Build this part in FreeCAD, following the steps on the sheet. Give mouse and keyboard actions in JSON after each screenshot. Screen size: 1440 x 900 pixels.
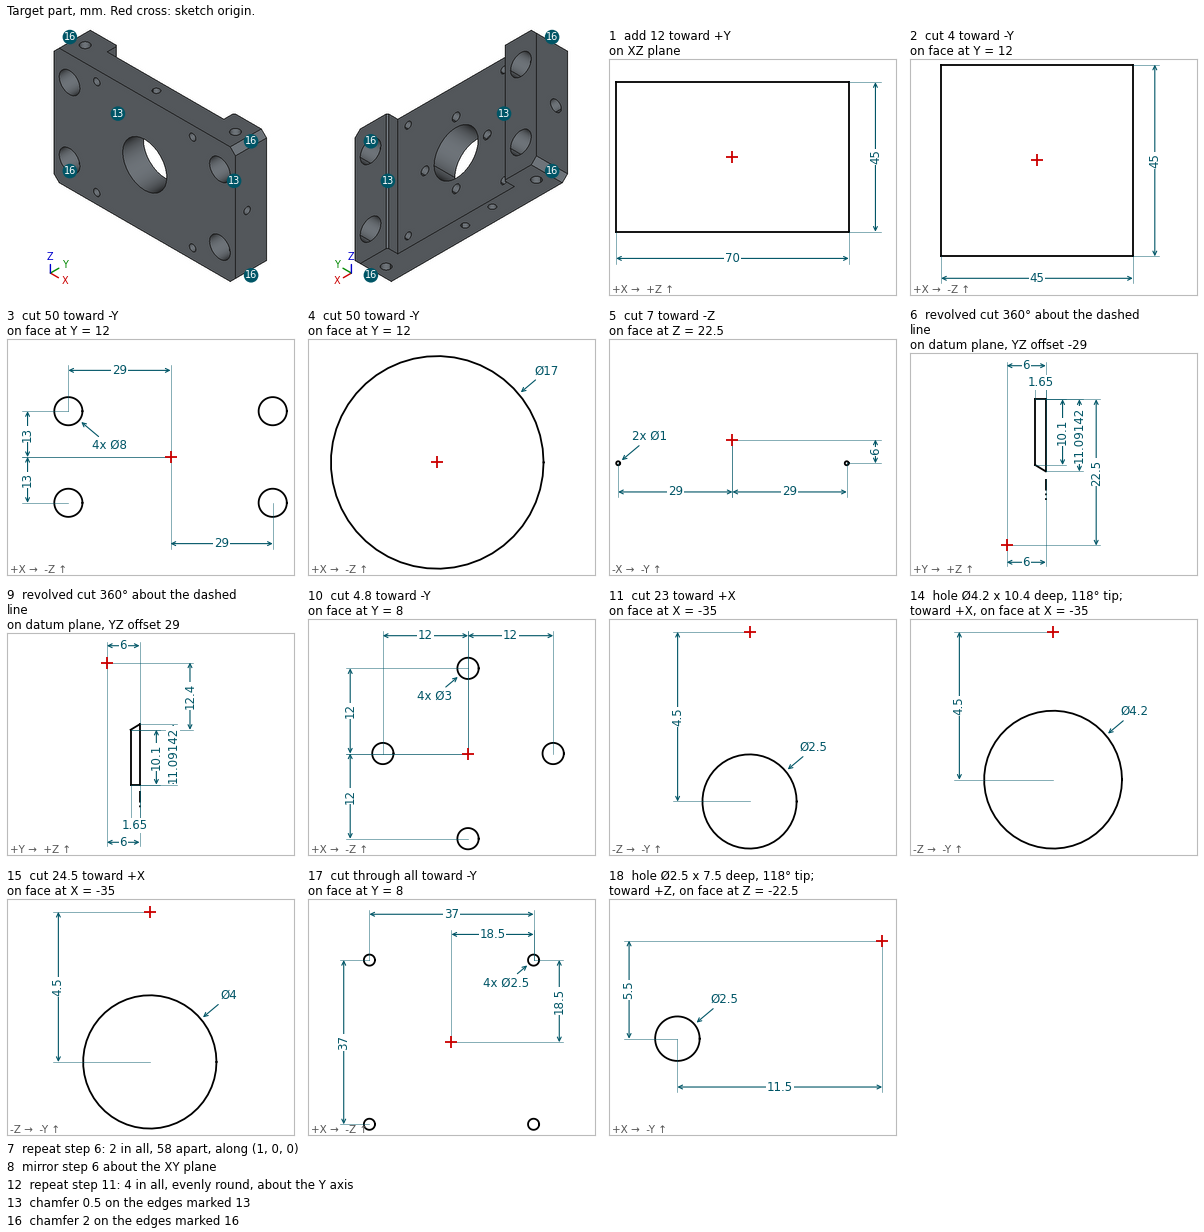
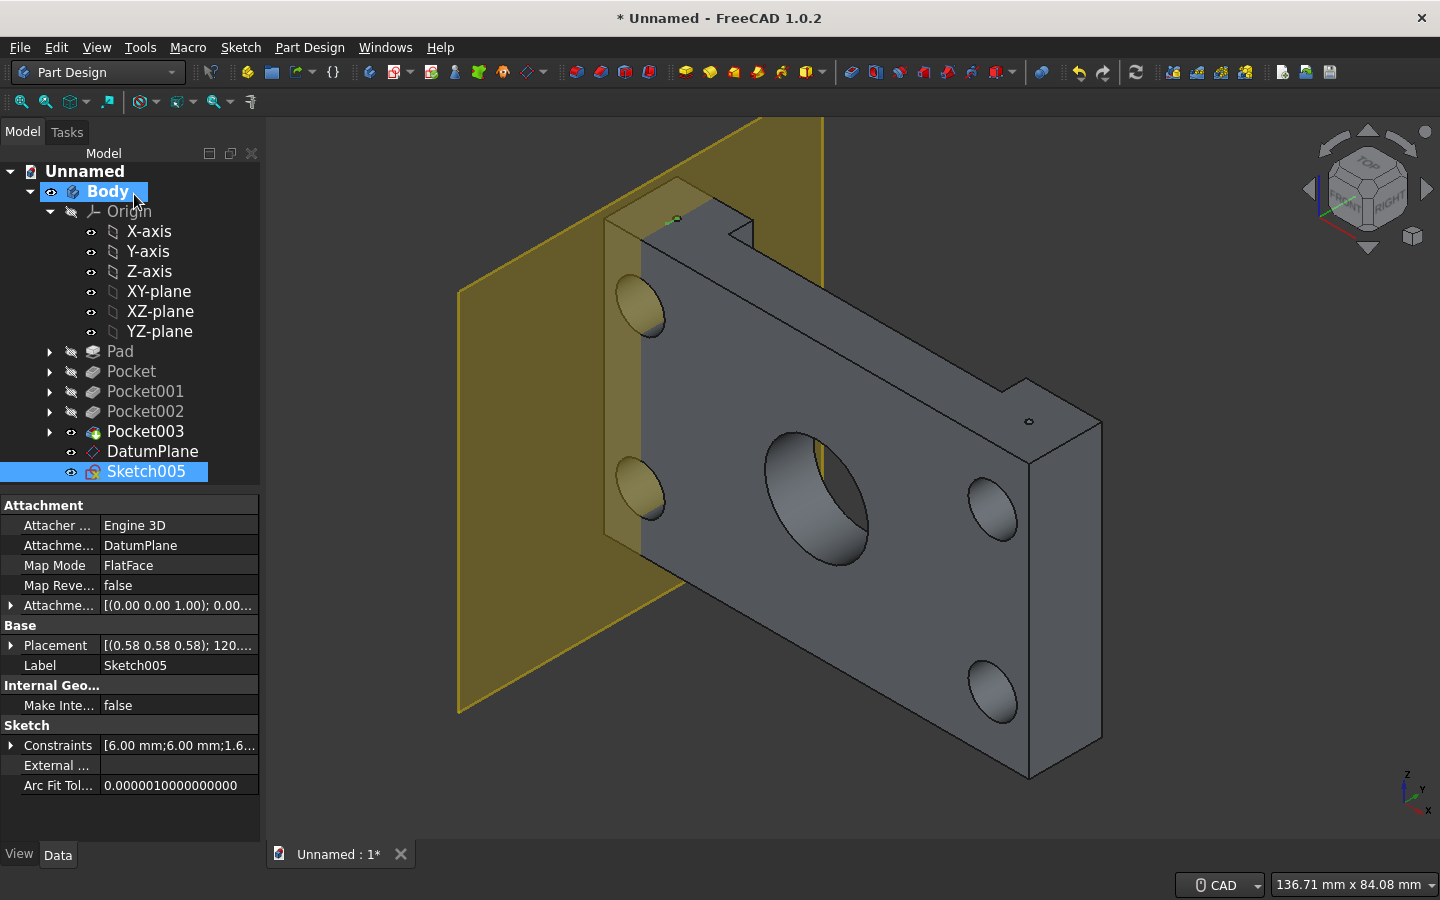
{"action": "left_click", "coordinate": [900, 72]}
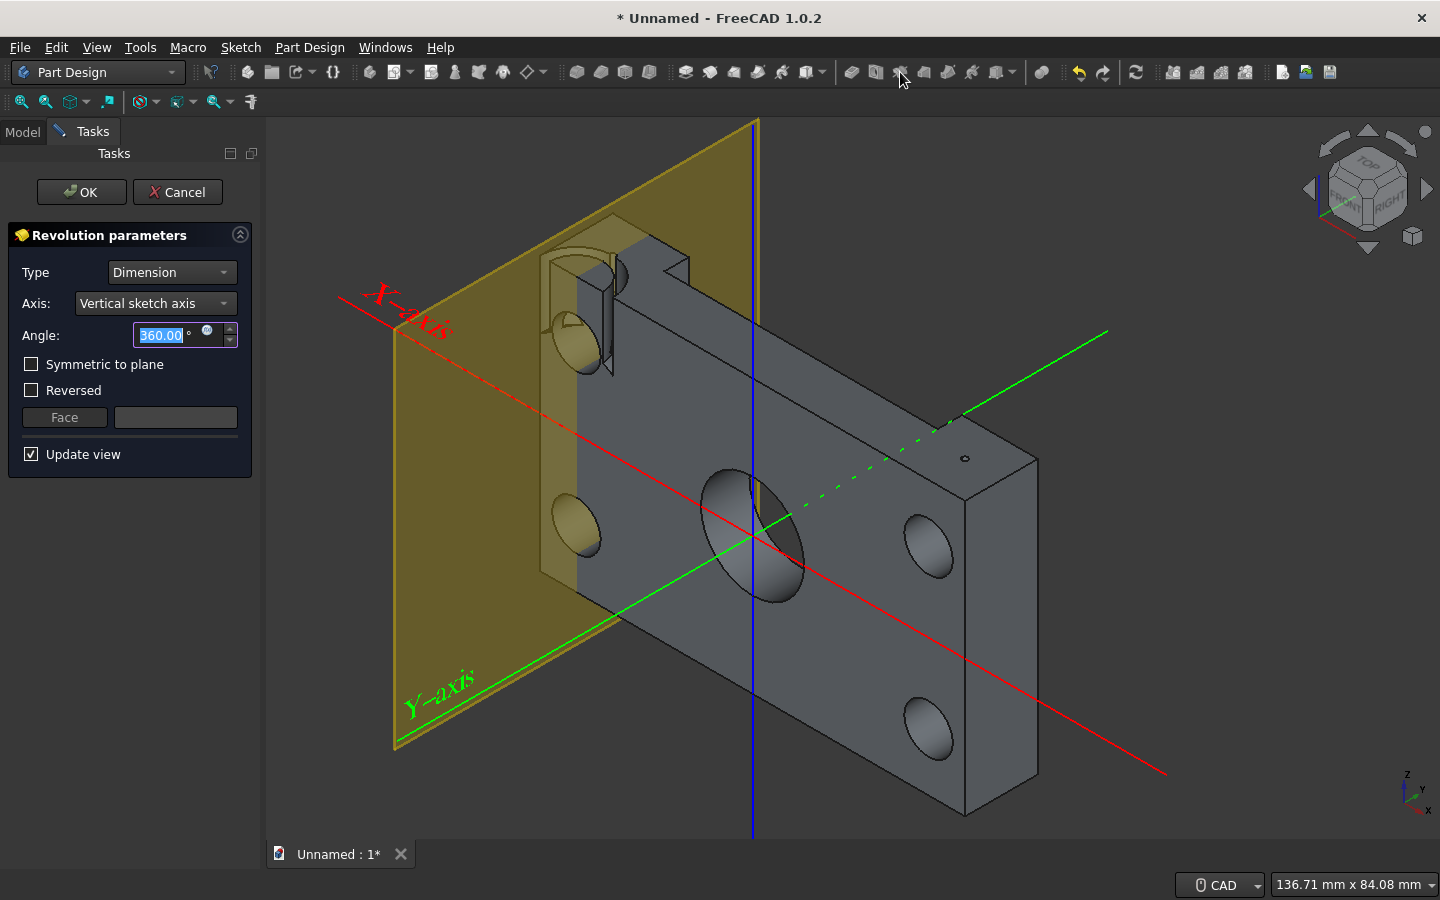
{"action": "left_click", "coordinate": [156, 304]}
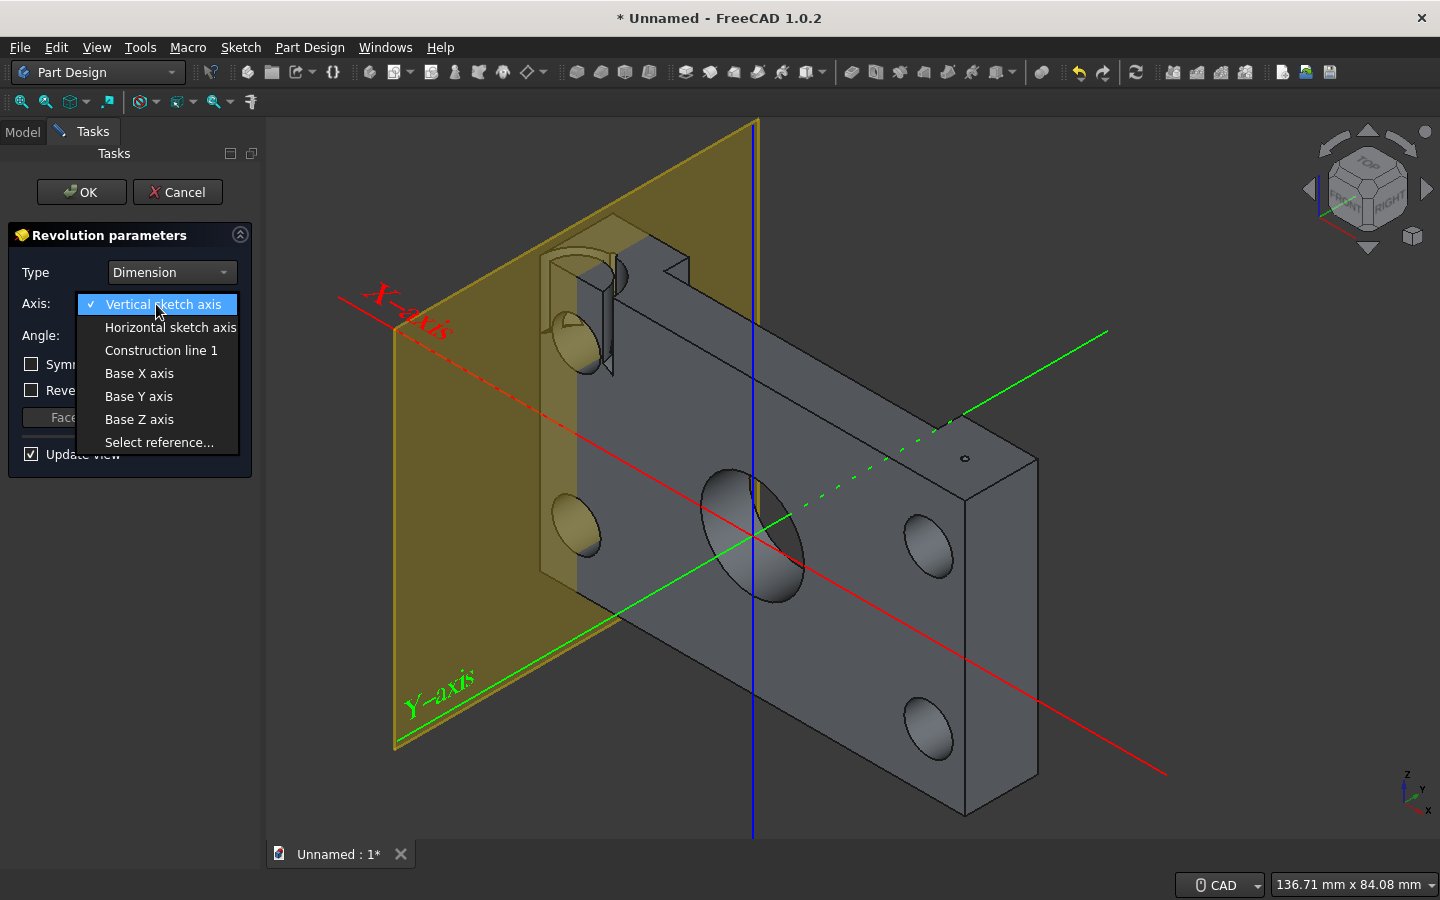
{"action": "left_click", "coordinate": [156, 350]}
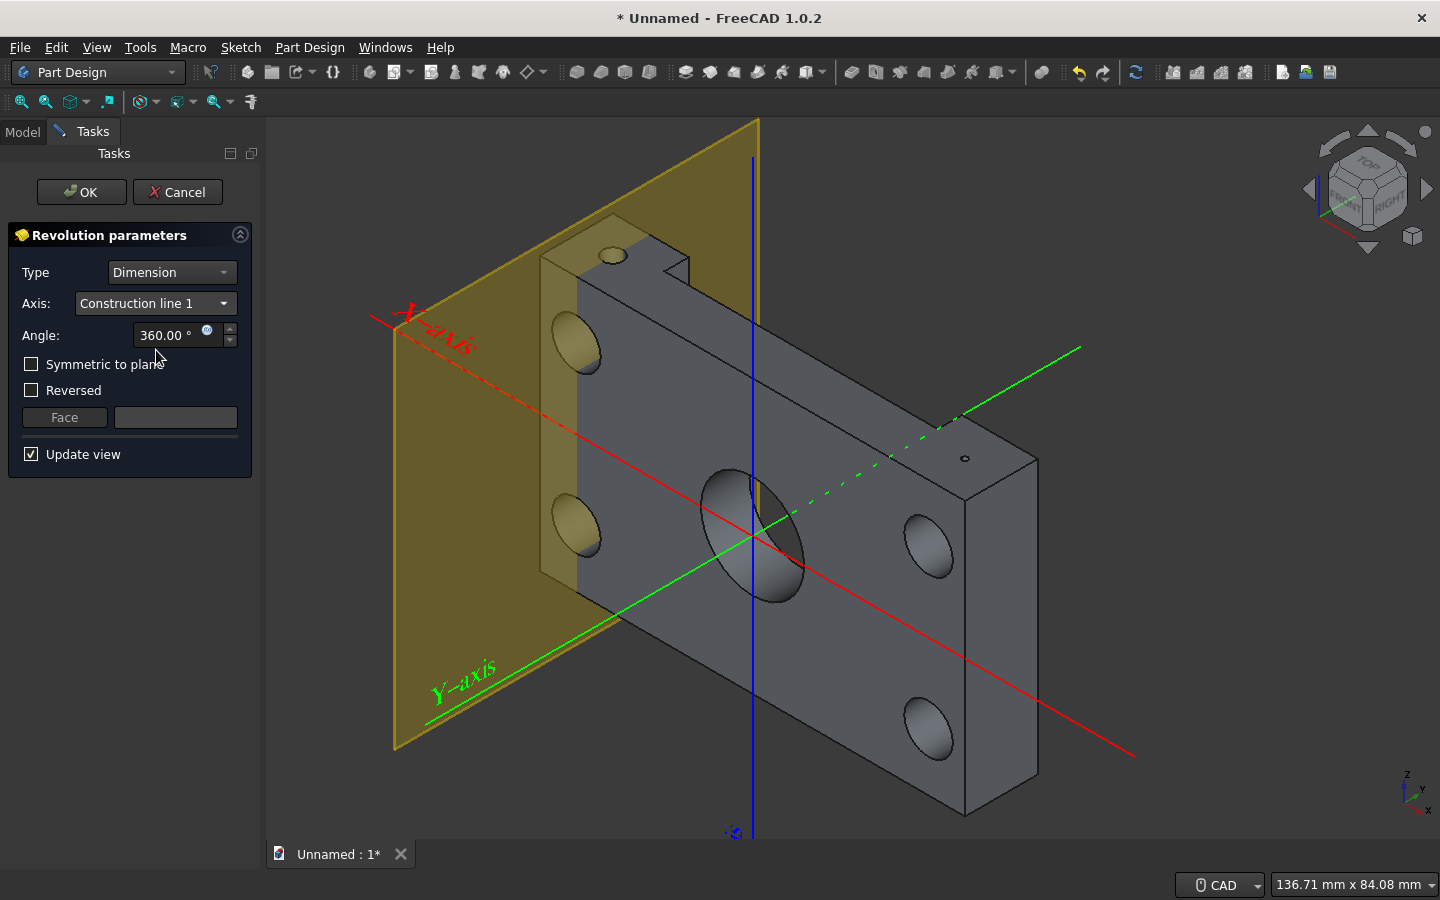
{"action": "left_click", "coordinate": [82, 192]}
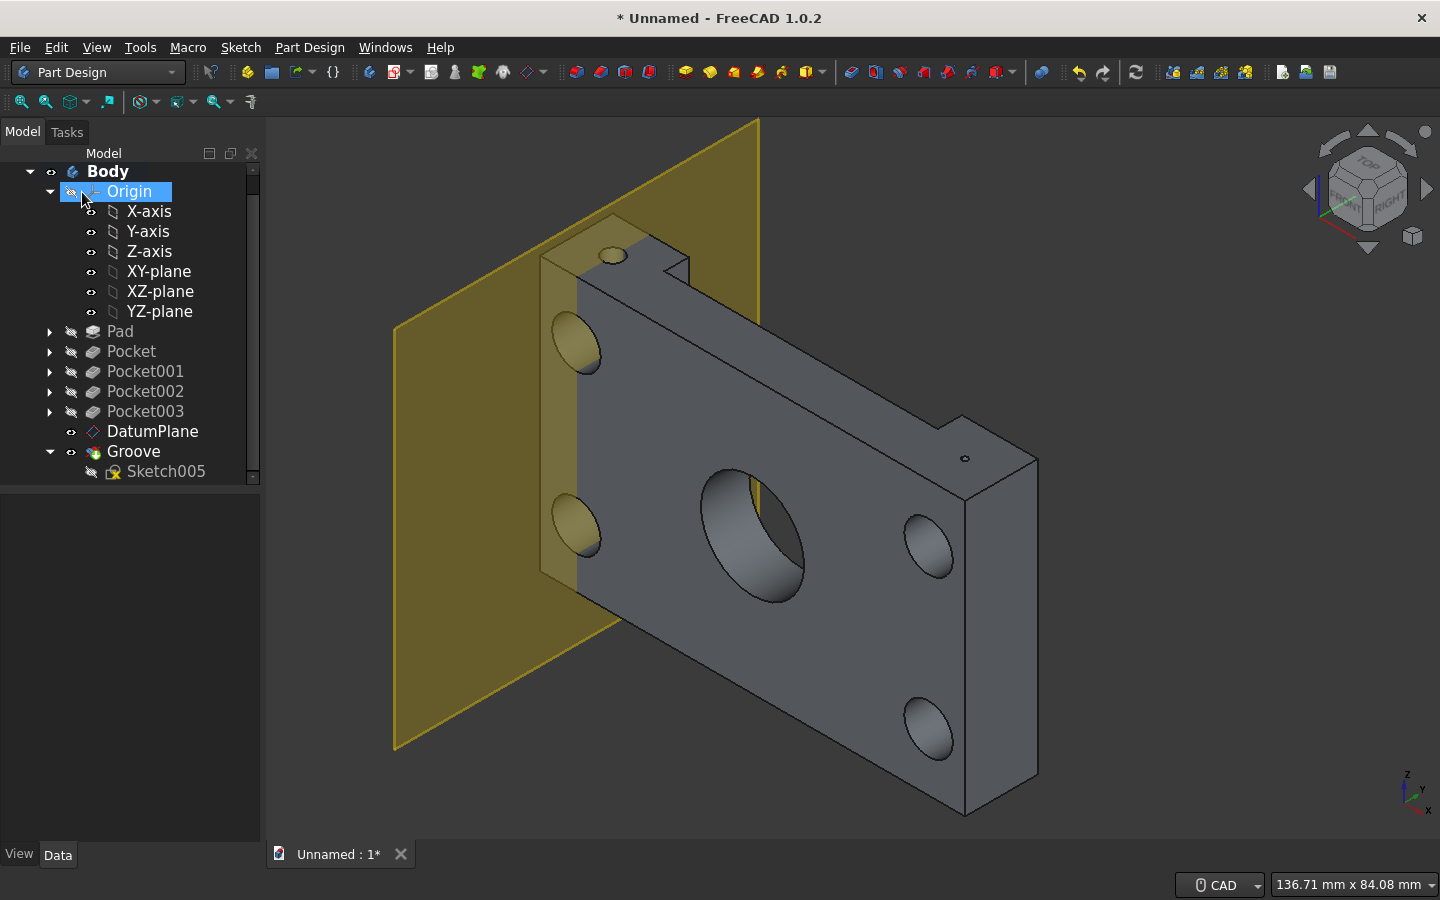
{"action": "left_click", "coordinate": [116, 432]}
{"action": "key", "text": "space"}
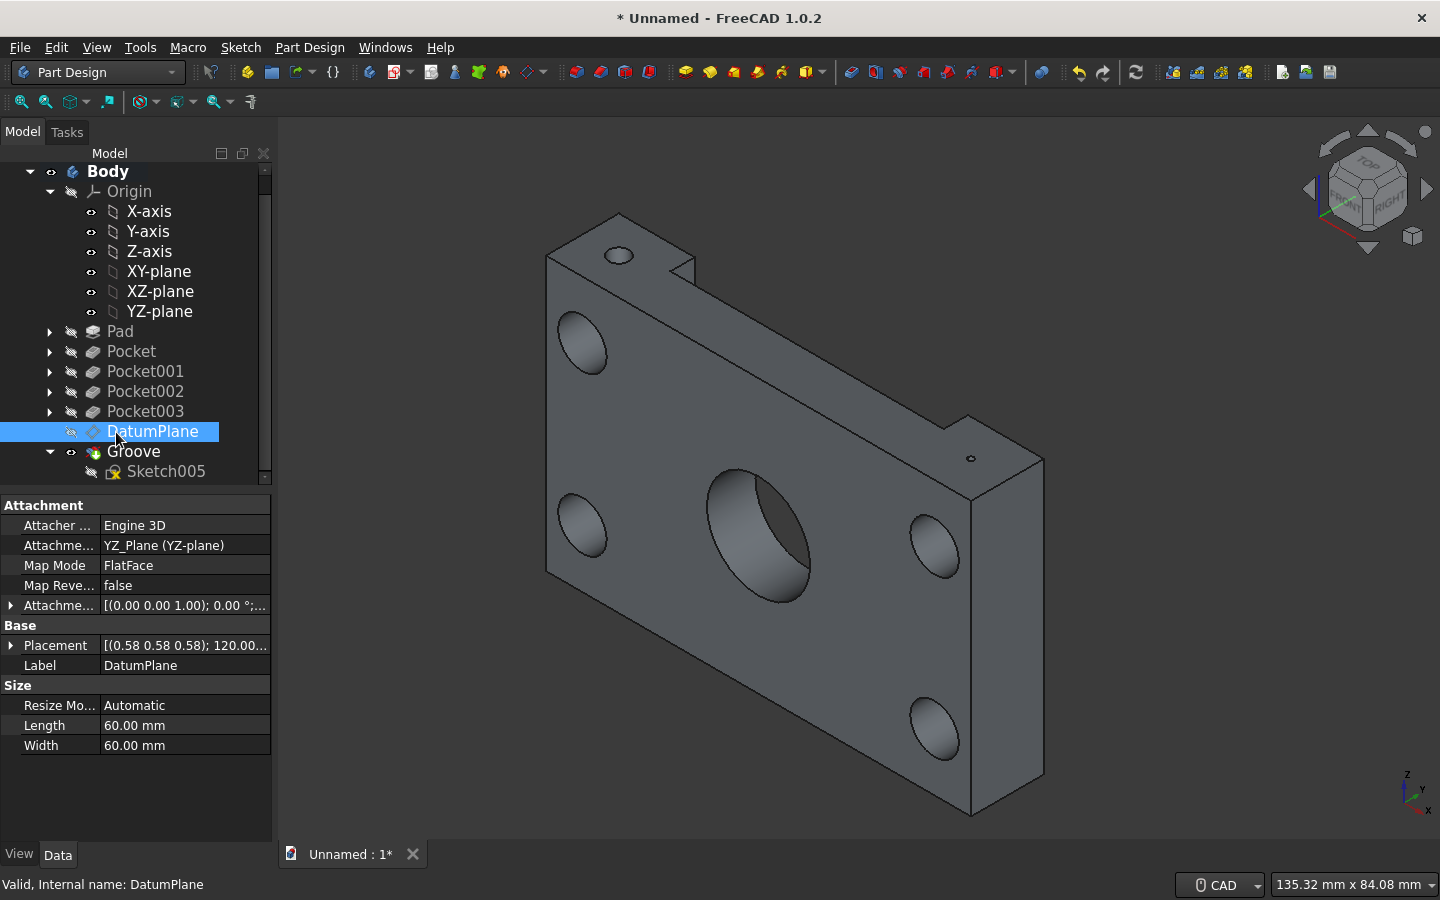
{"action": "left_click", "coordinate": [116, 452]}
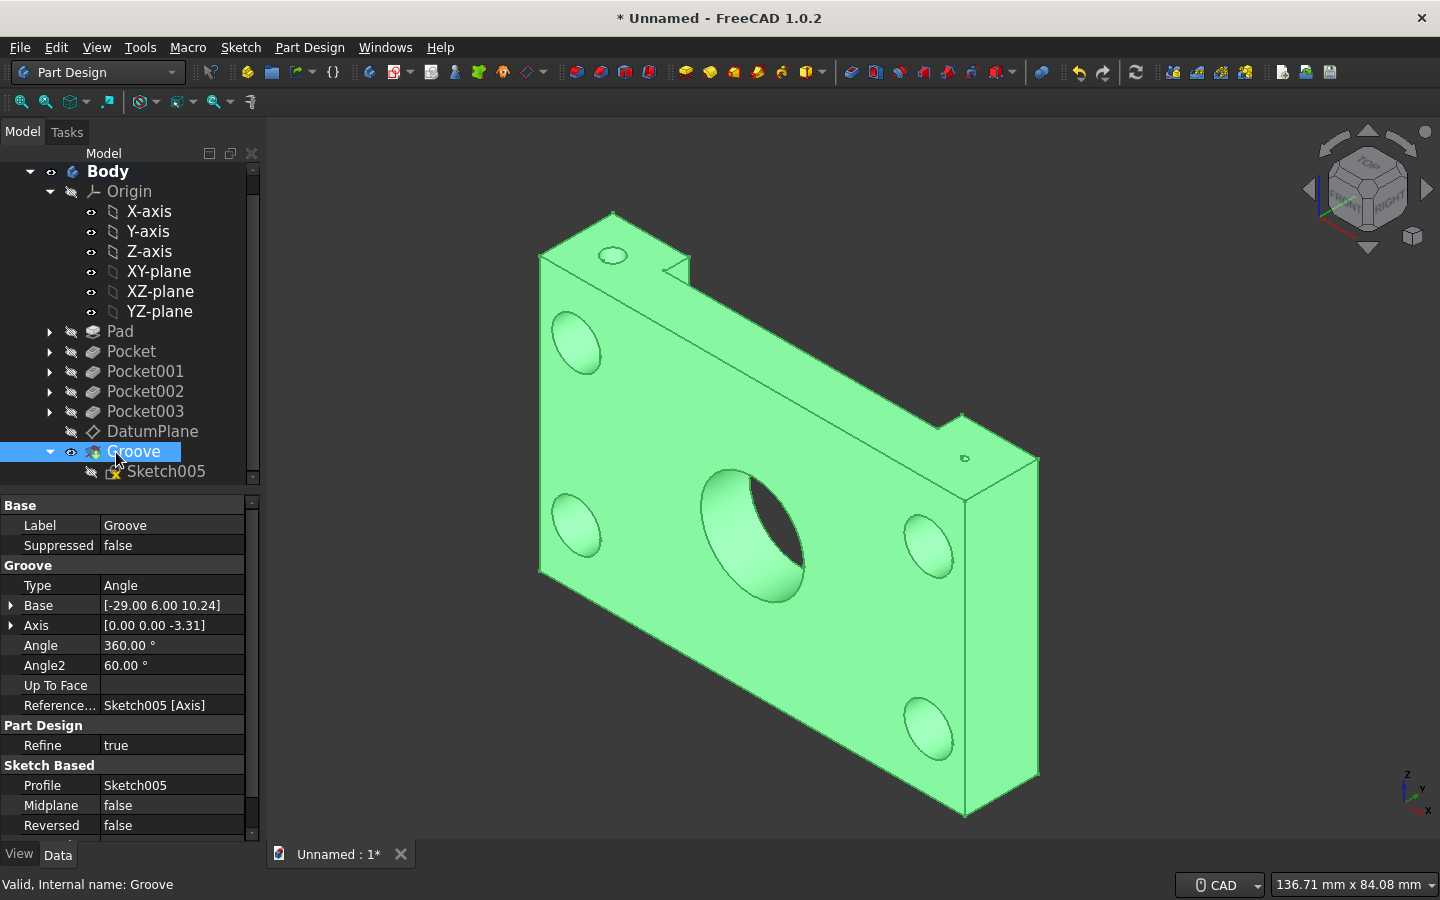
{"action": "left_click", "coordinate": [1198, 72]}